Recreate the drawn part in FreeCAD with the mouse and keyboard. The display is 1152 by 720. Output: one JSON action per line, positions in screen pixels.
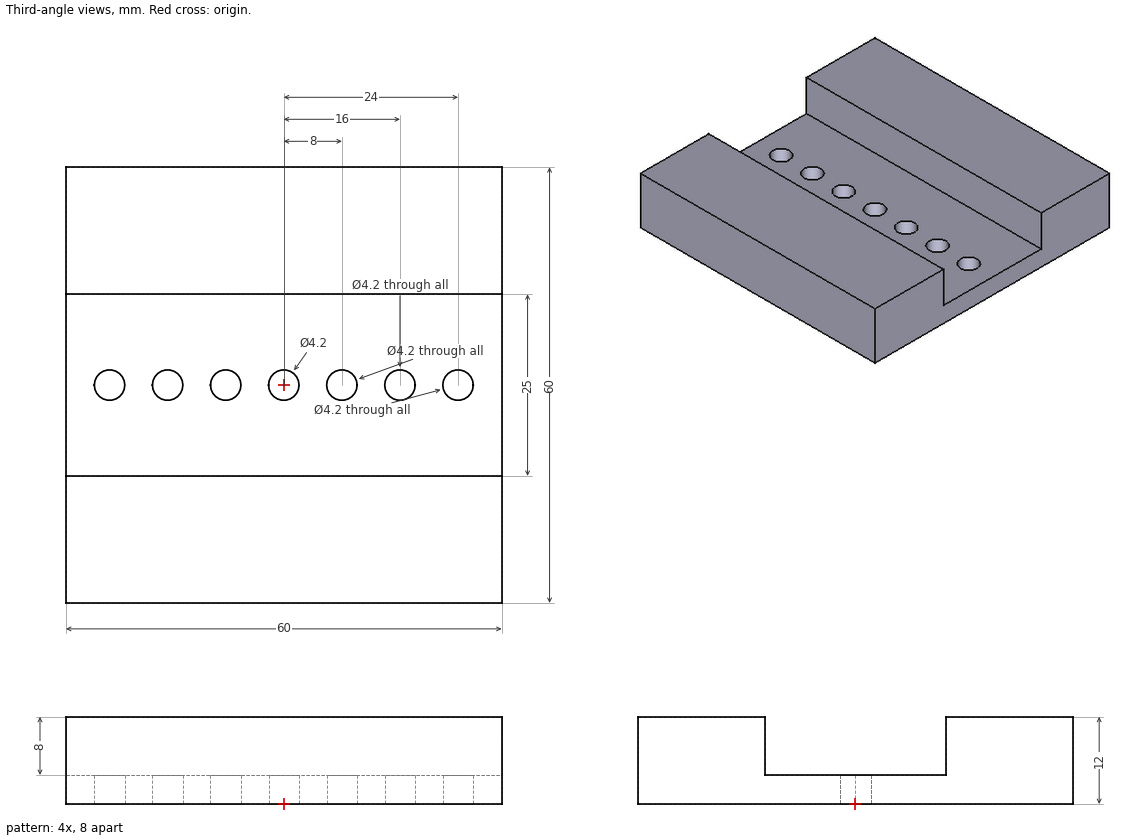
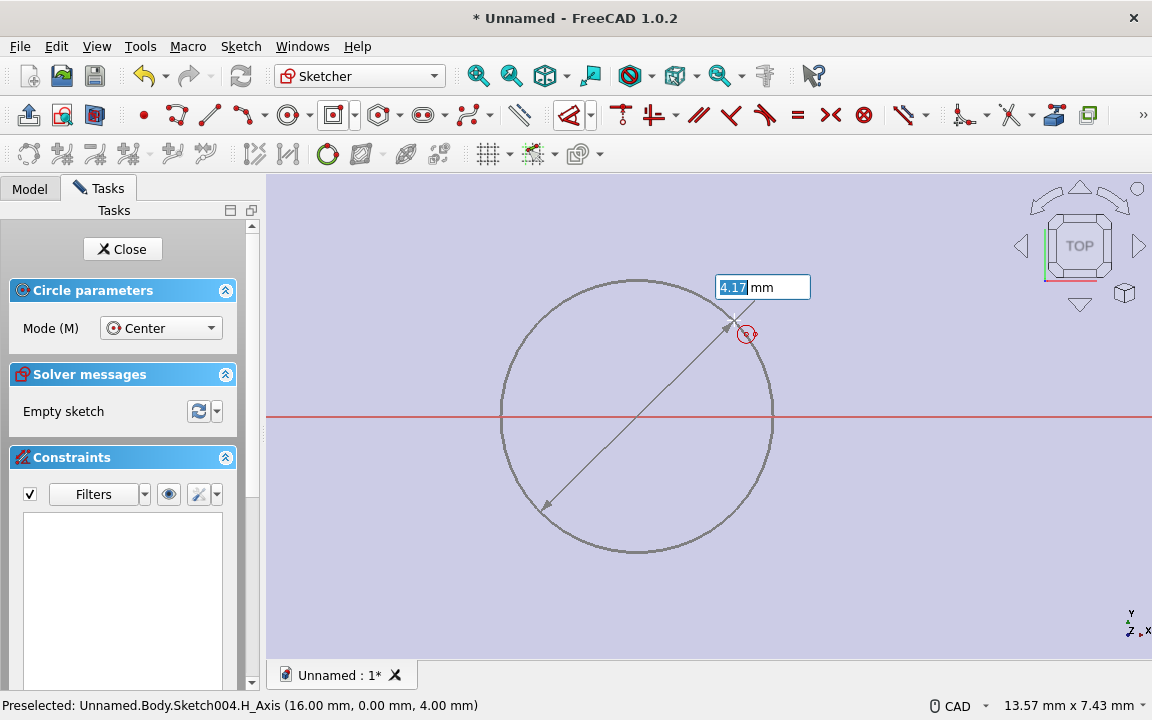
{"action": "type", "text": "4.2"}
{"action": "key", "text": "Return"}
{"action": "key", "text": "Escape"}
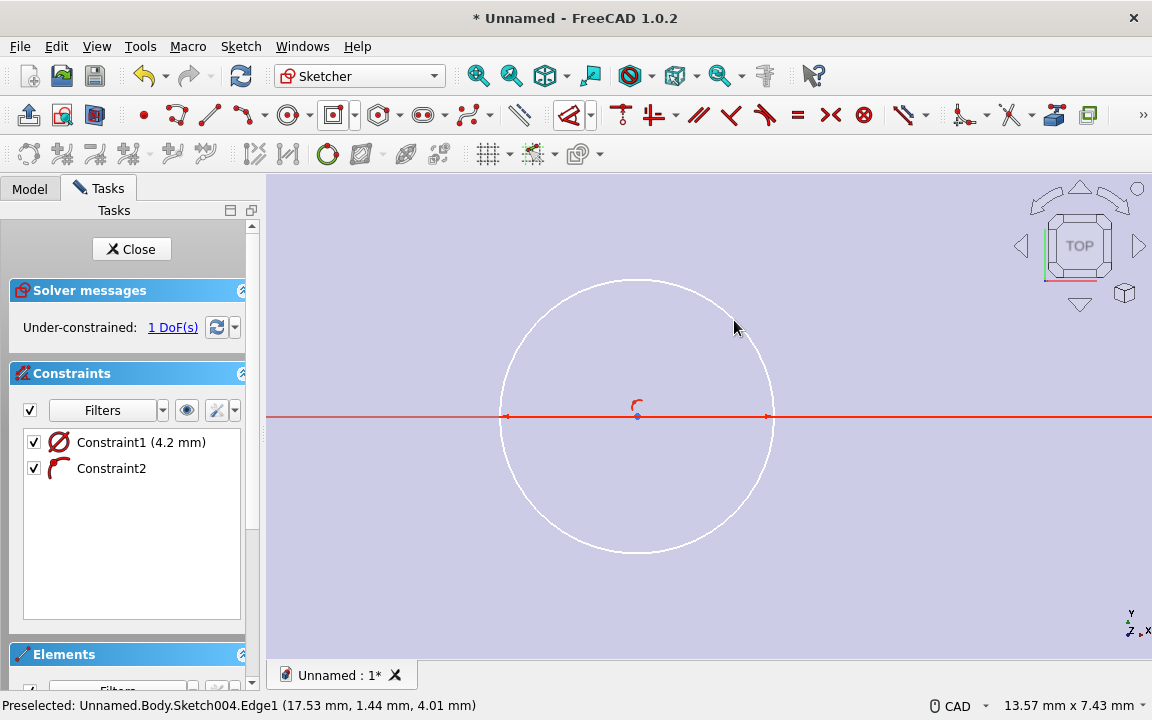
{"action": "left_click", "coordinate": [637, 416]}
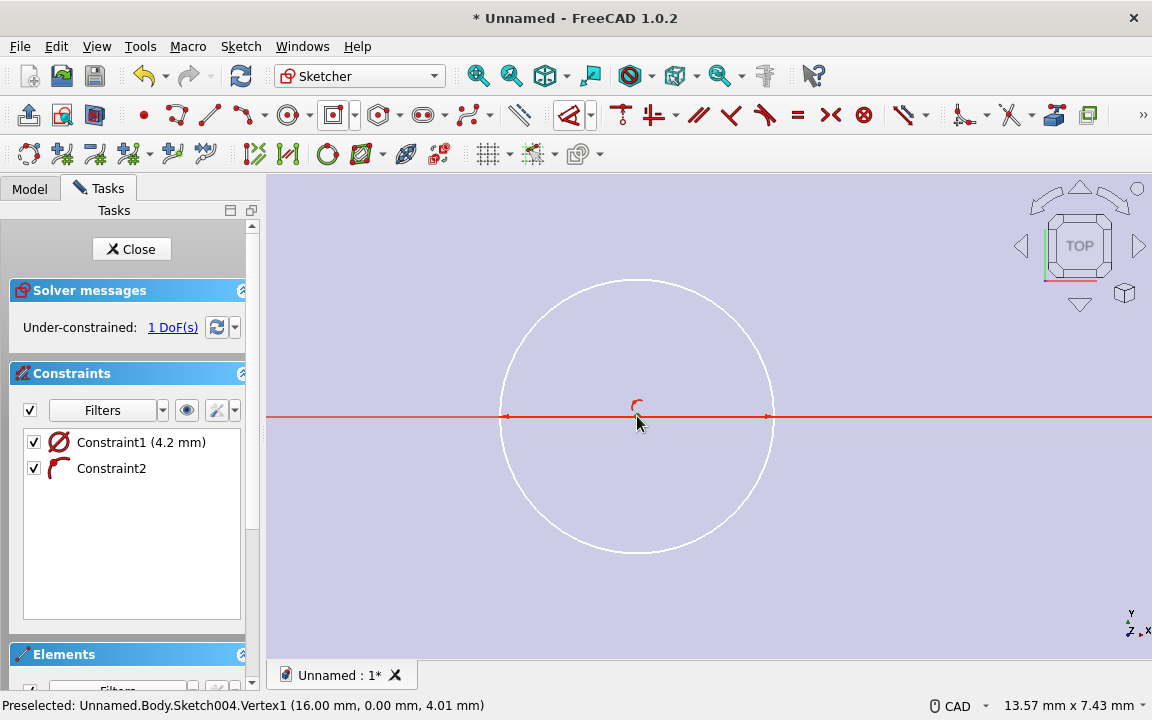
{"action": "left_click", "coordinate": [590, 116]}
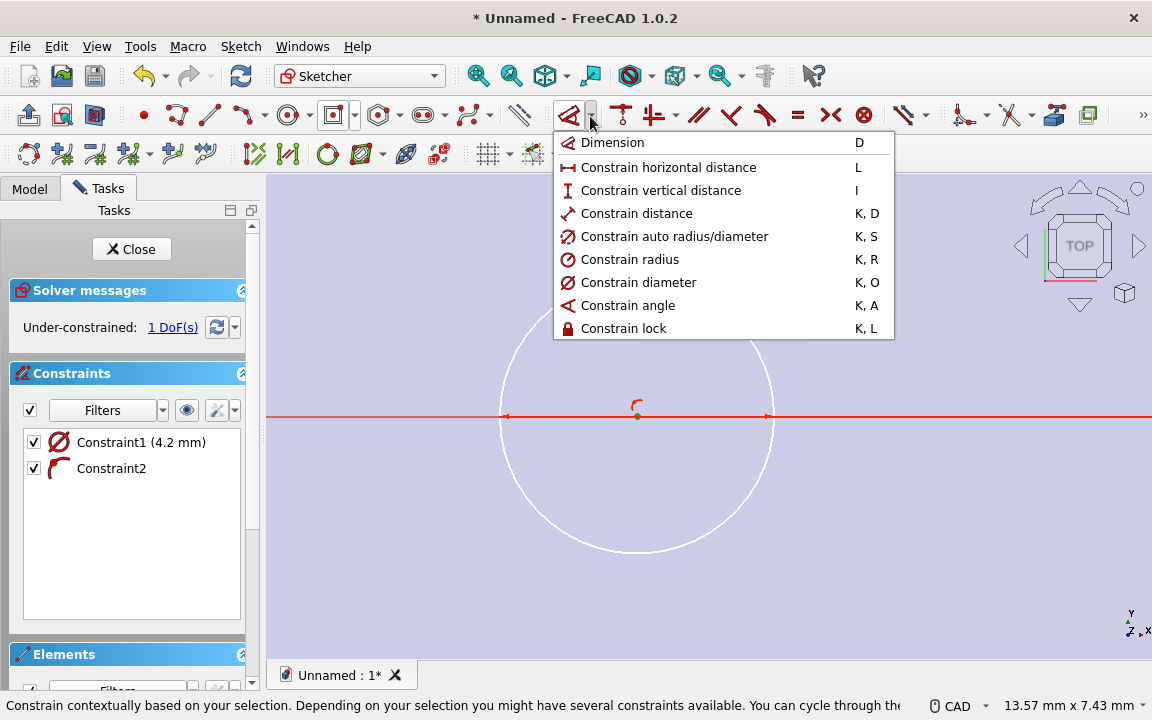
{"action": "left_click", "coordinate": [724, 168]}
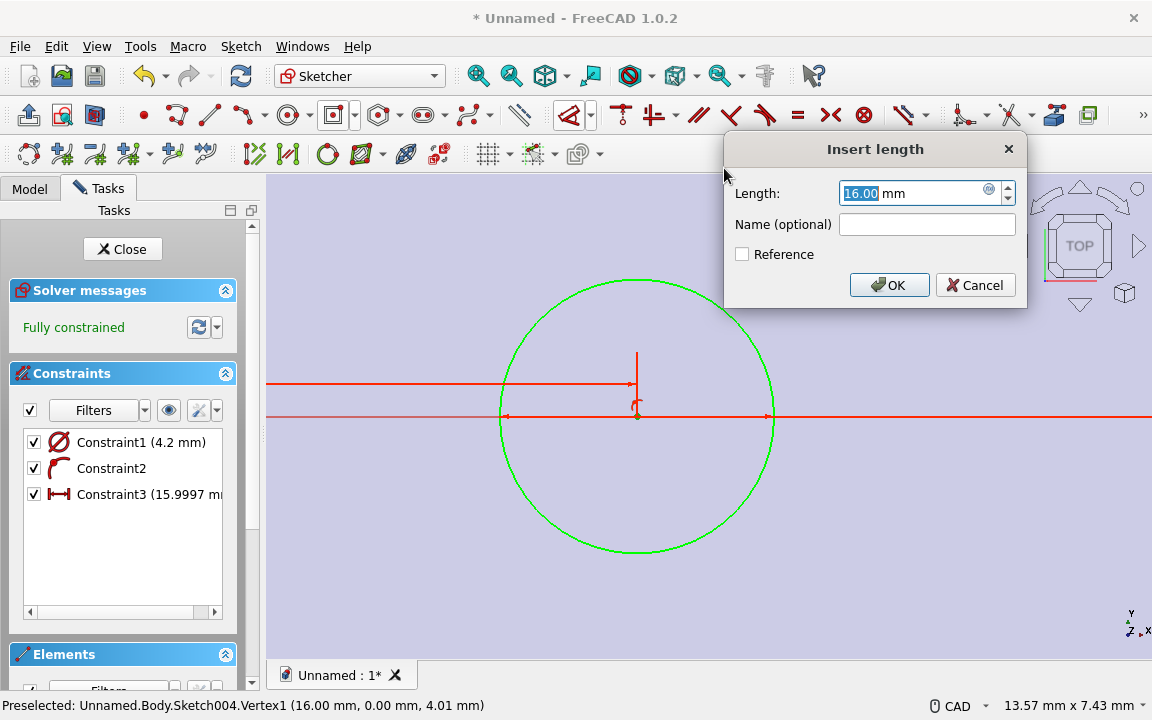
{"action": "type", "text": "16"}
{"action": "key", "text": "Return"}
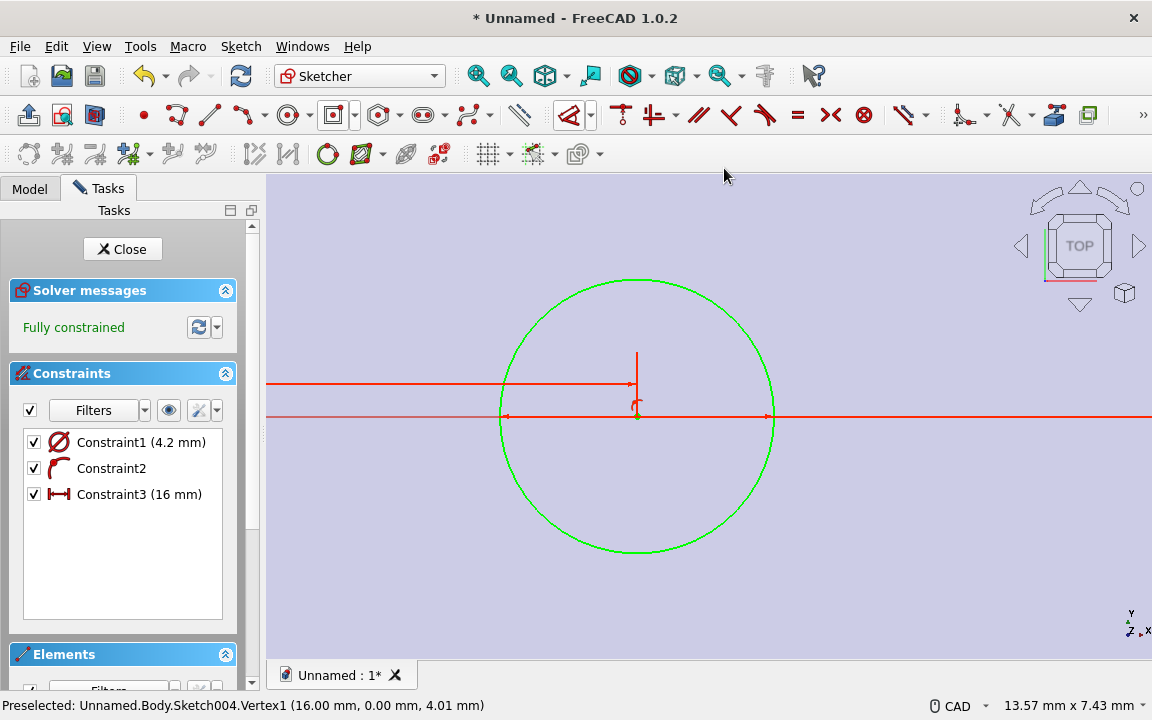
{"action": "left_click", "coordinate": [123, 249]}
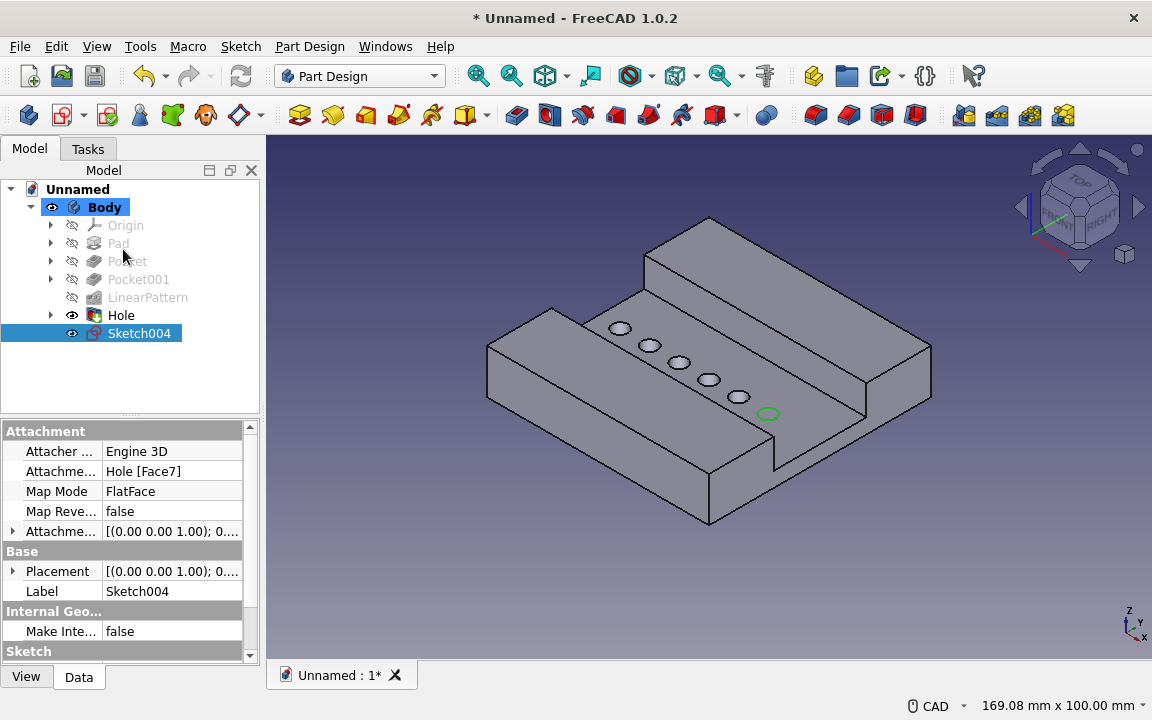
{"action": "left_click", "coordinate": [550, 116]}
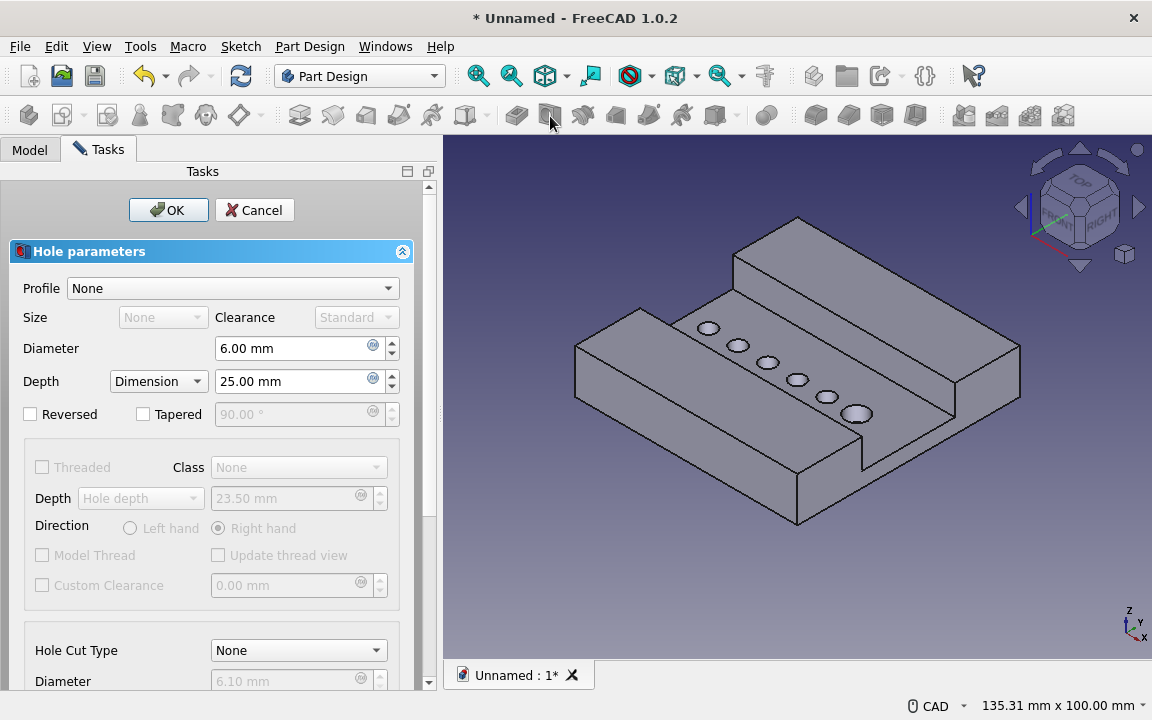
{"action": "triple_click", "coordinate": [300, 348]}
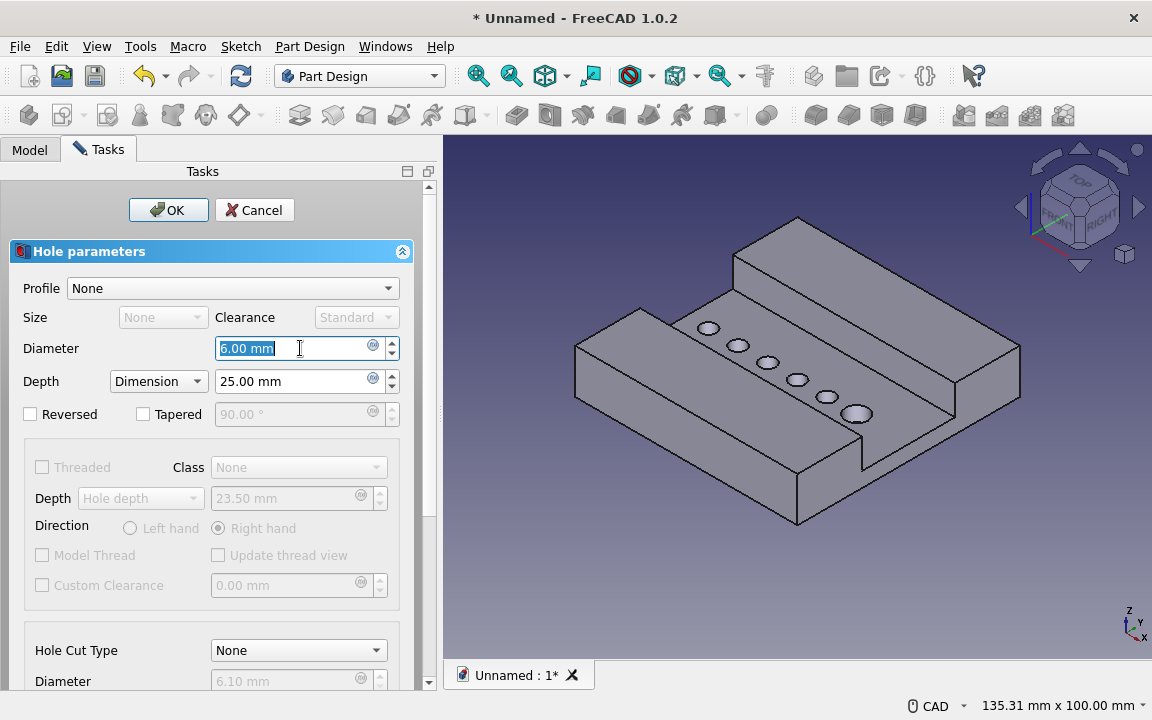
{"action": "type", "text": "4.2"}
{"action": "key", "text": "Tab"}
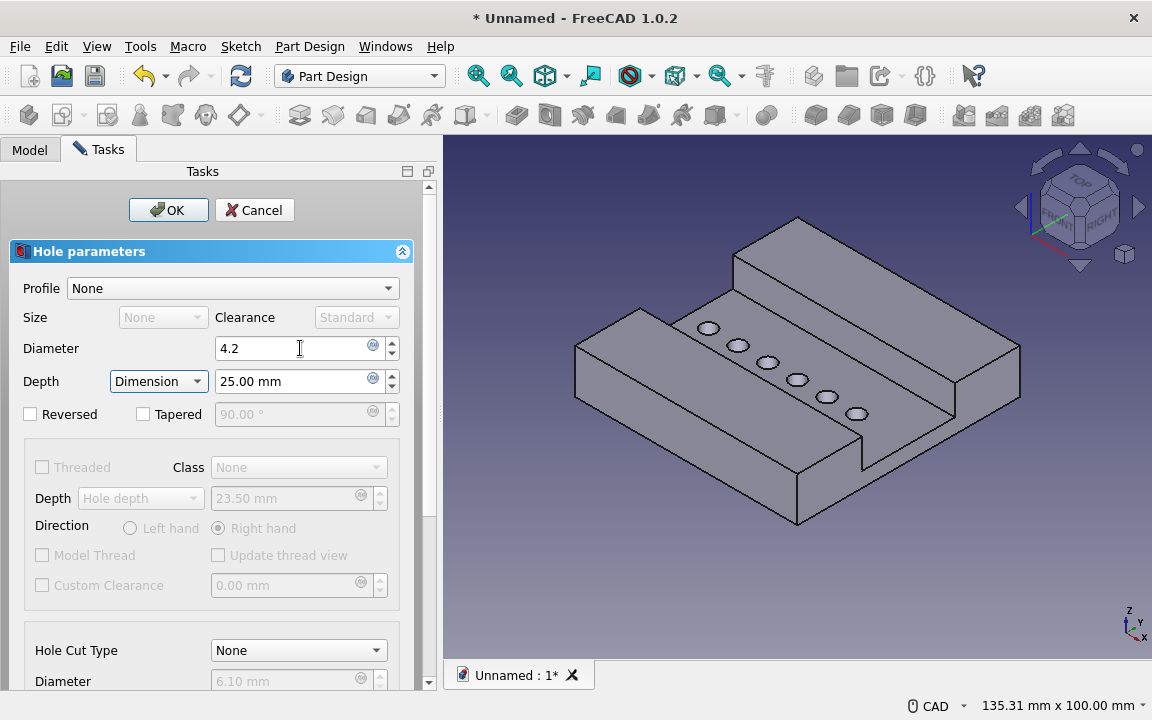
{"action": "left_click", "coordinate": [160, 382]}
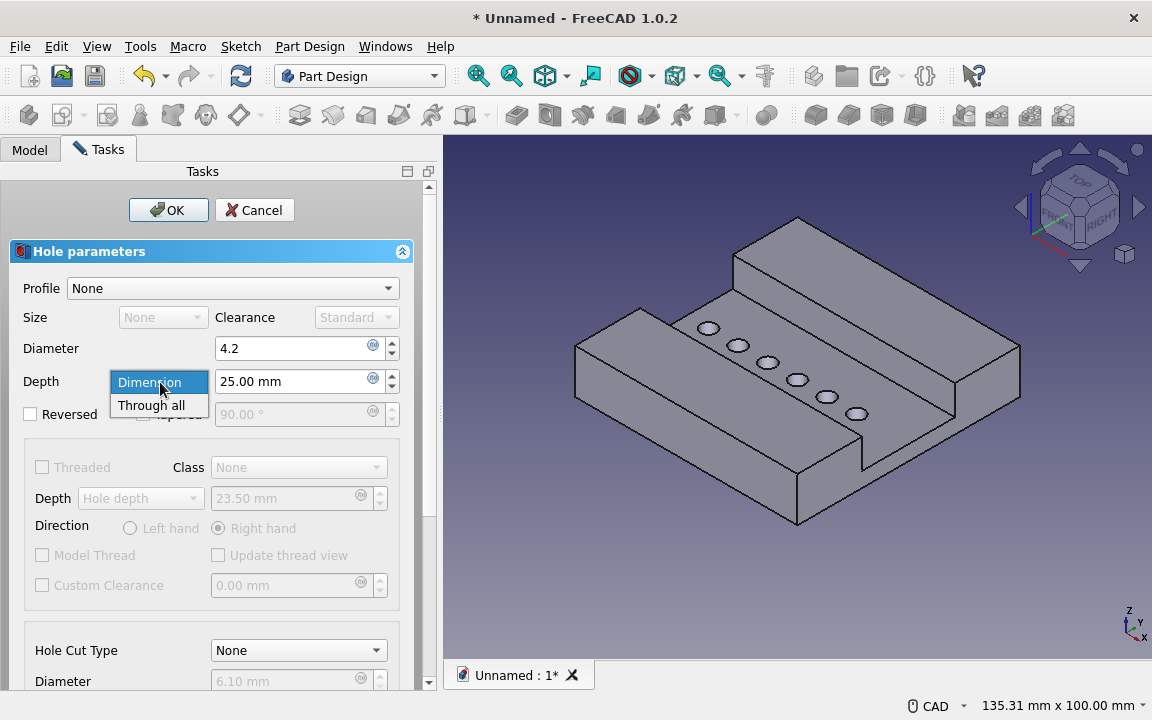
{"action": "left_click", "coordinate": [158, 406]}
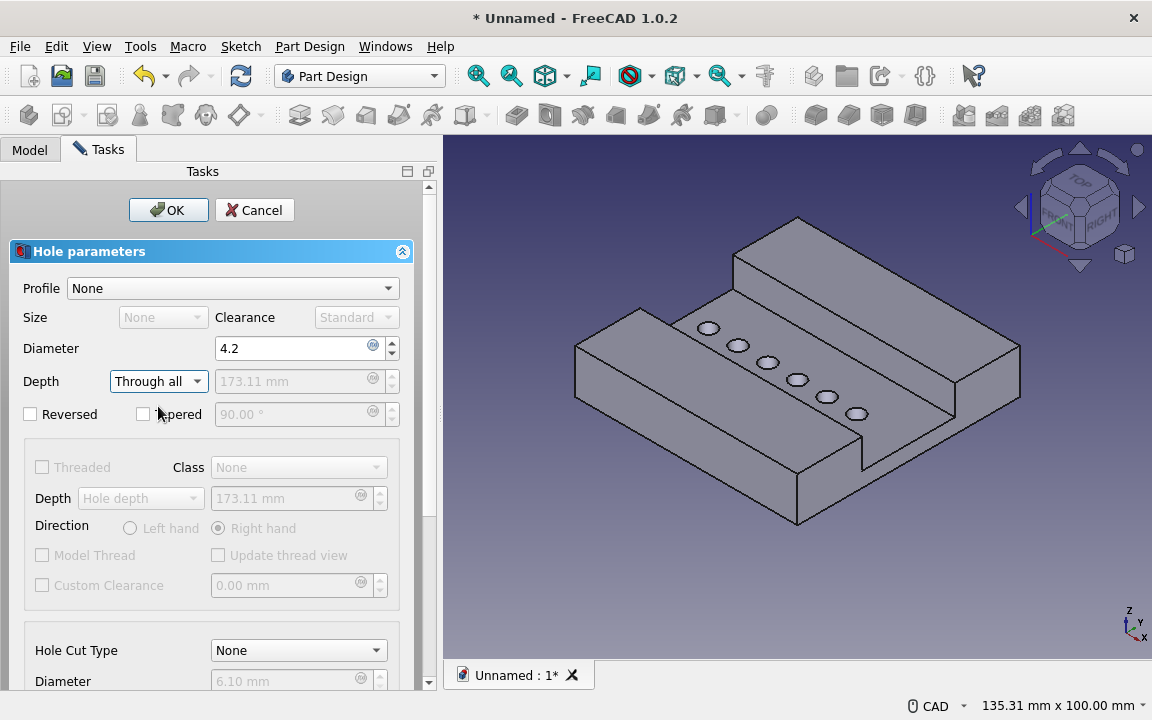
{"action": "left_click", "coordinate": [169, 210]}